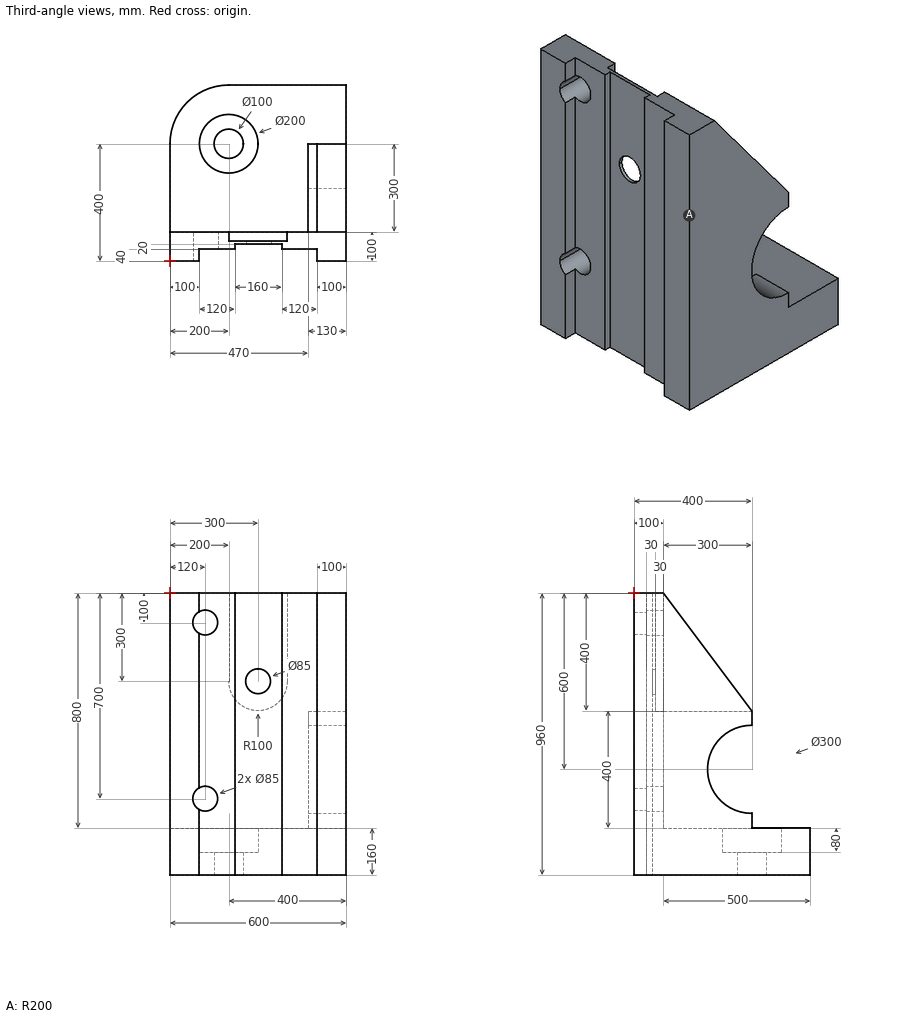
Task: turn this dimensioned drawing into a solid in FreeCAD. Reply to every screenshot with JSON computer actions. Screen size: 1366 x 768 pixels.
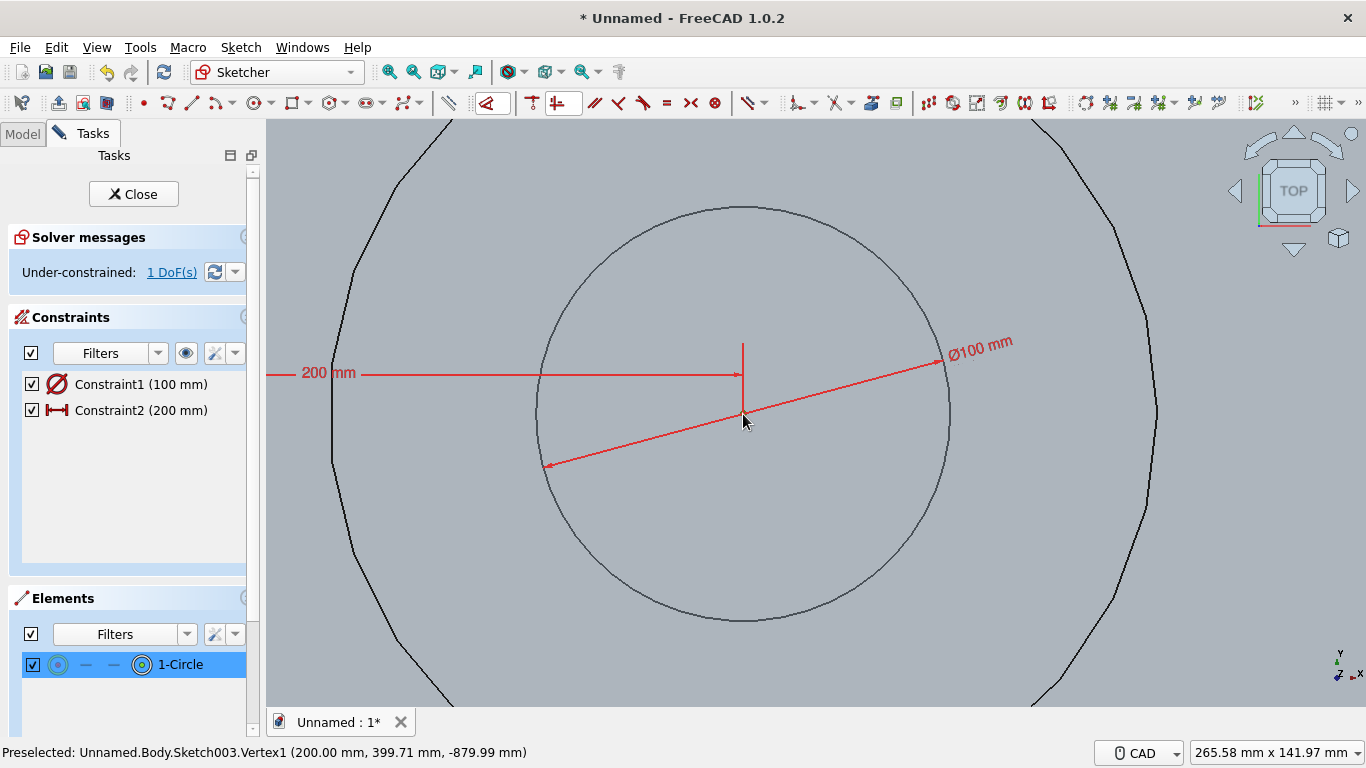
{"action": "left_click", "coordinate": [504, 104]}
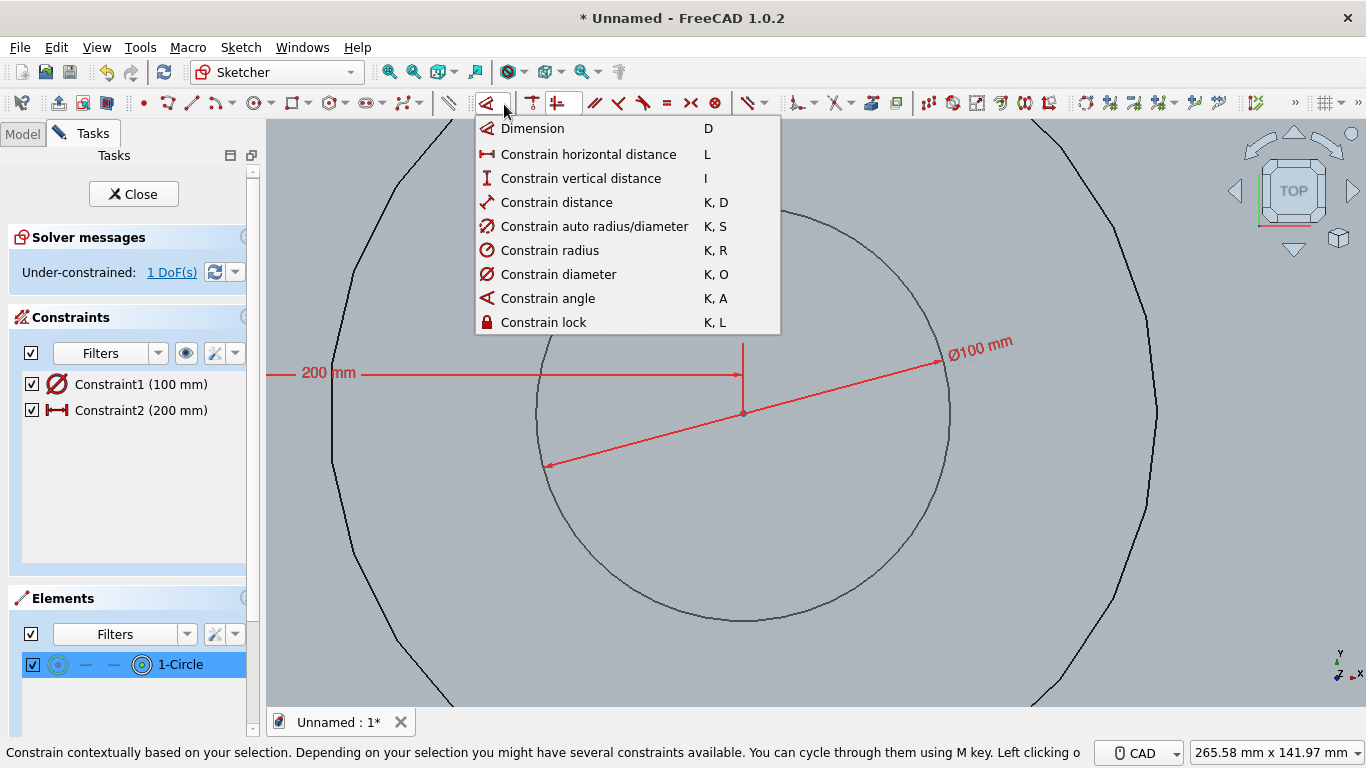
{"action": "left_click", "coordinate": [628, 178]}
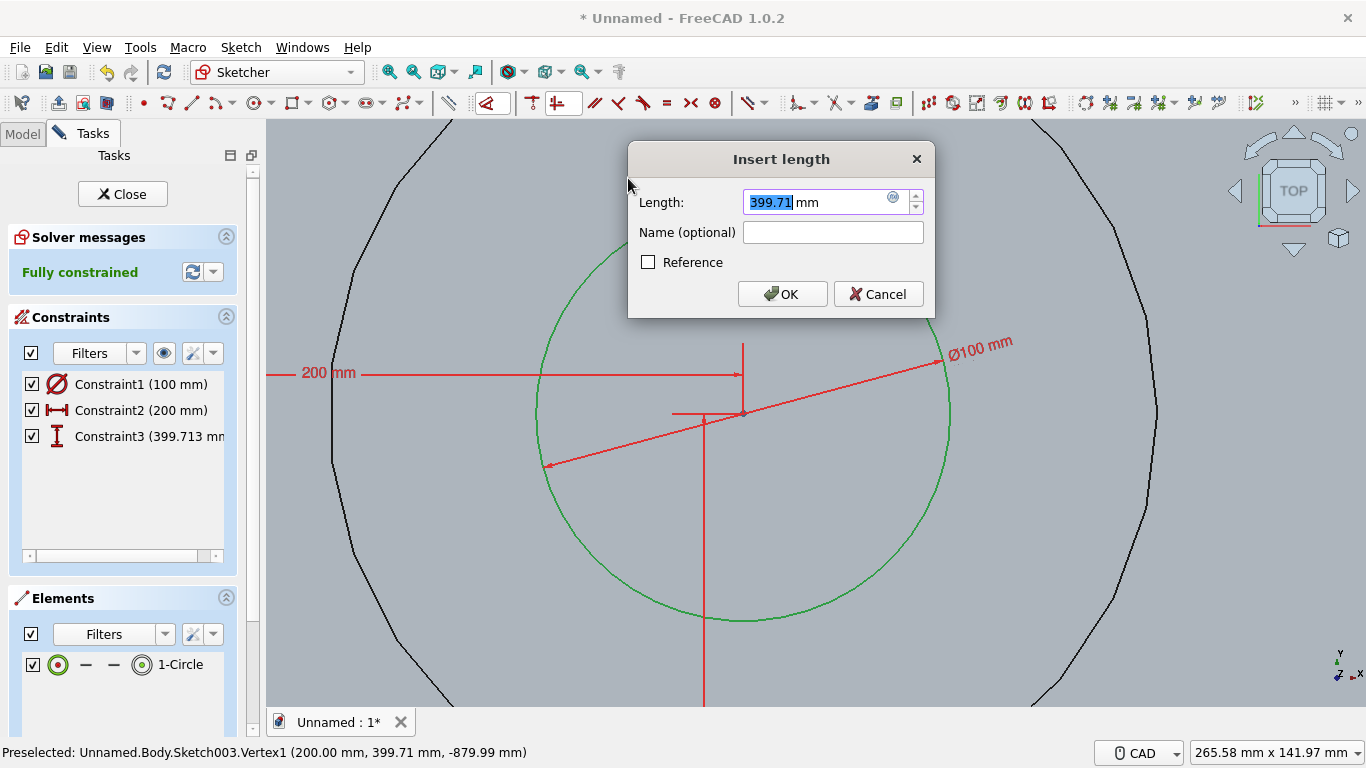
{"action": "type", "text": "400"}
{"action": "key", "text": "Return"}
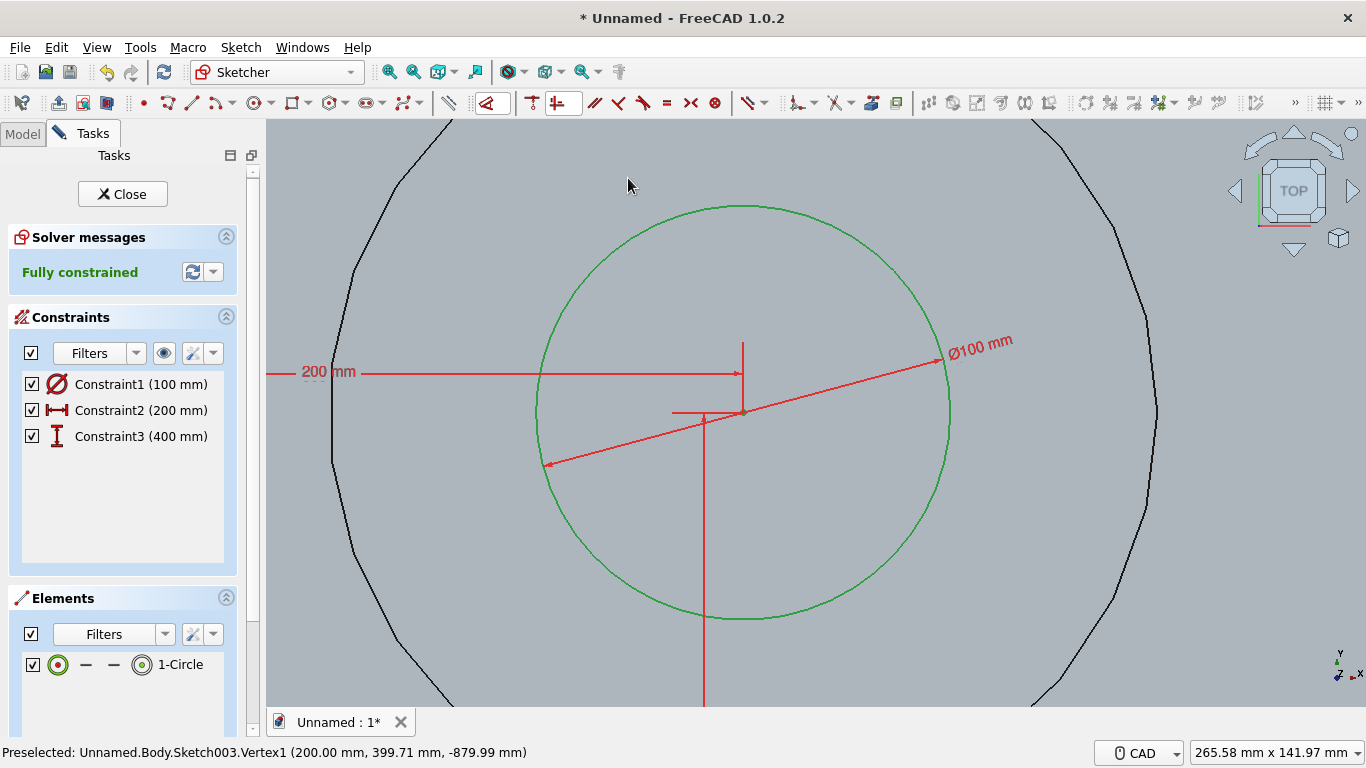
{"action": "left_click", "coordinate": [123, 194]}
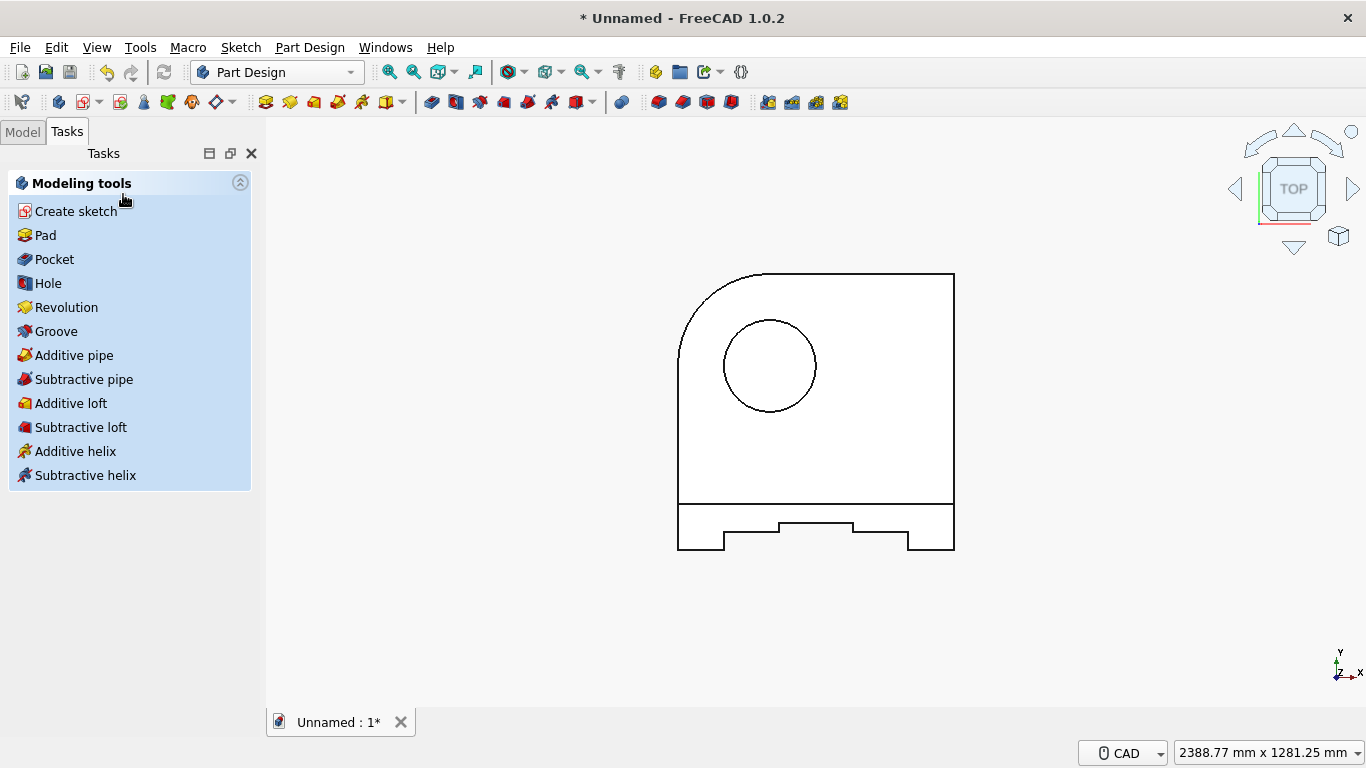
{"action": "left_click", "coordinate": [432, 102]}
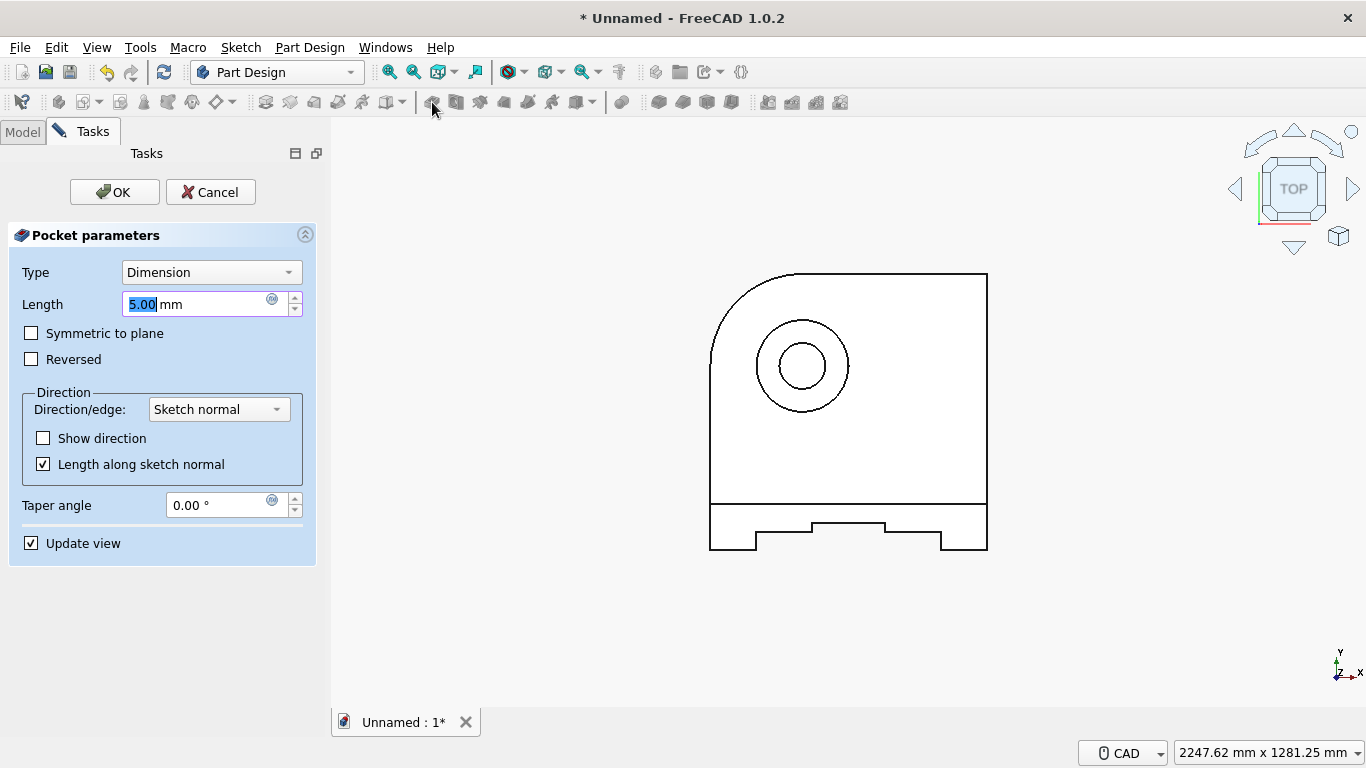
{"action": "left_click", "coordinate": [212, 272]}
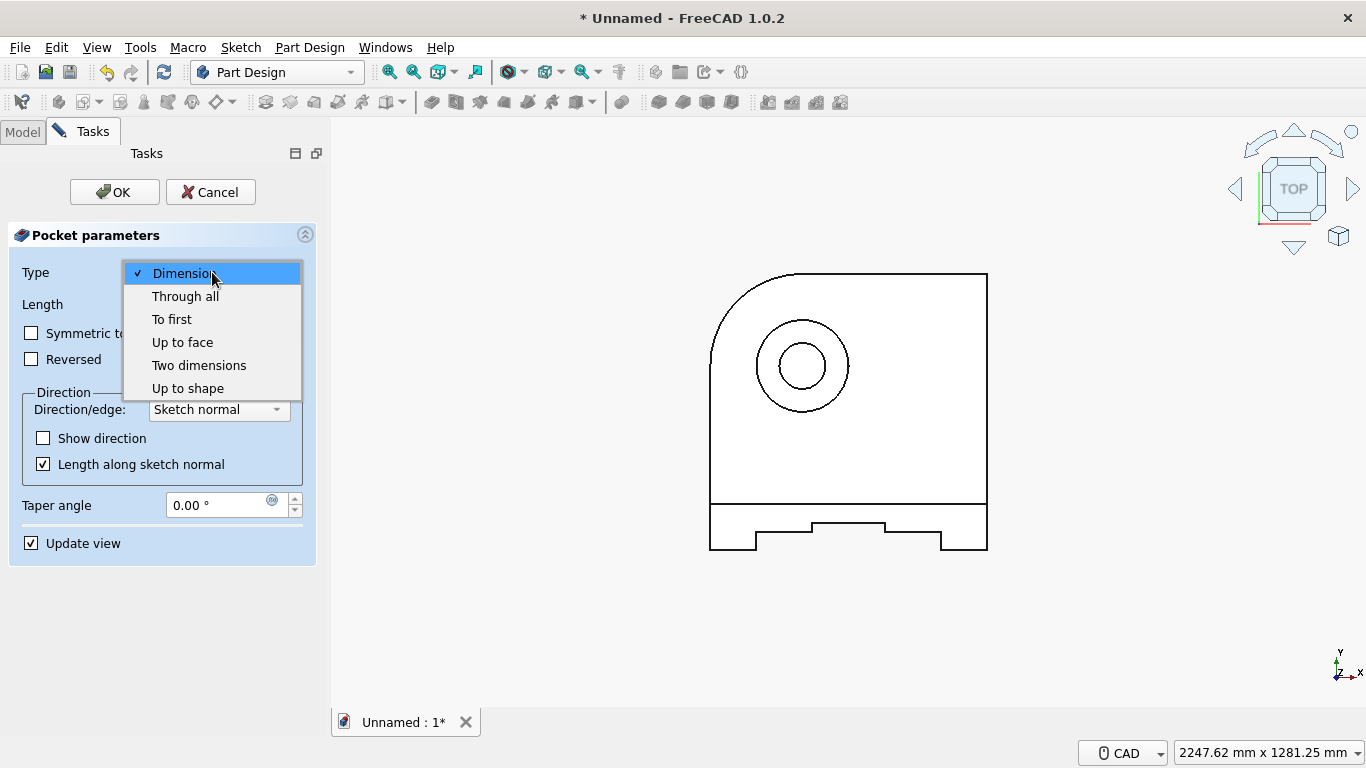
{"action": "left_click", "coordinate": [212, 296]}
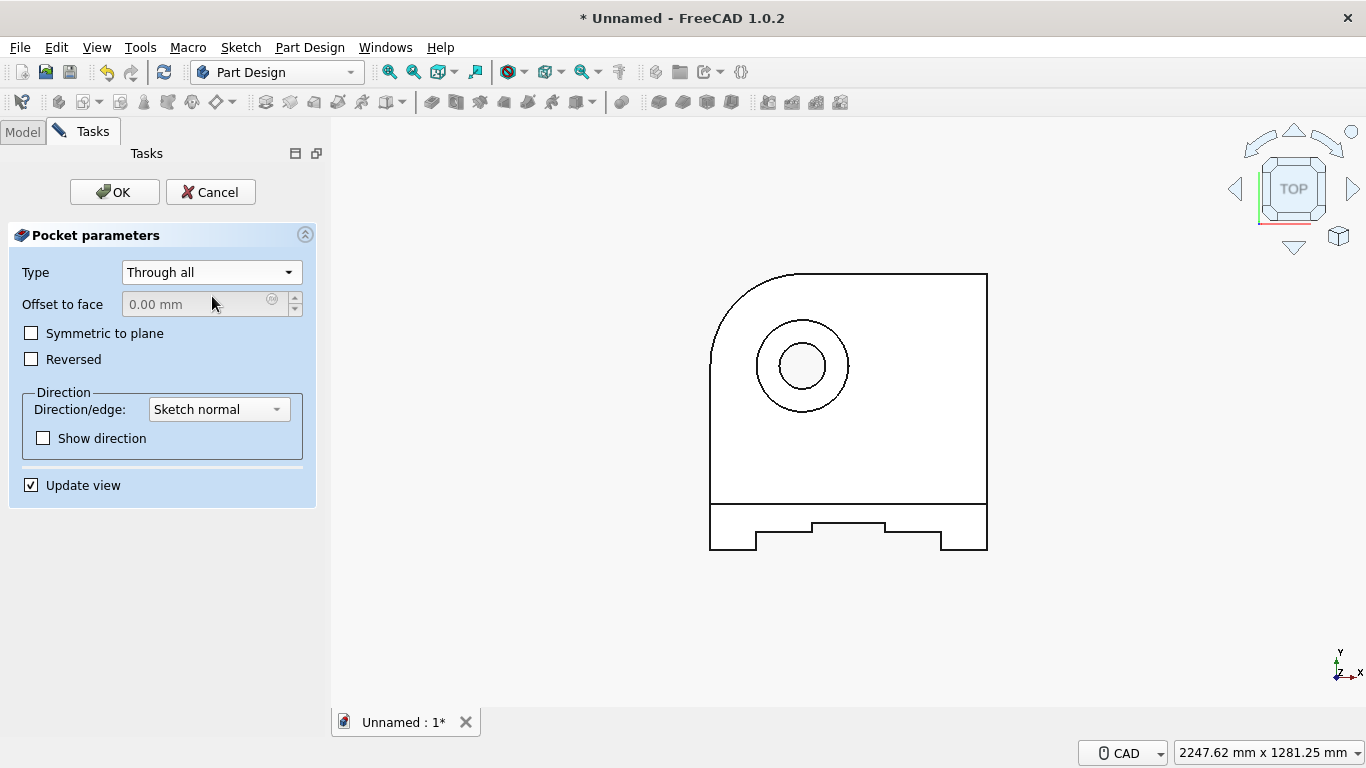
{"action": "left_click", "coordinate": [115, 192]}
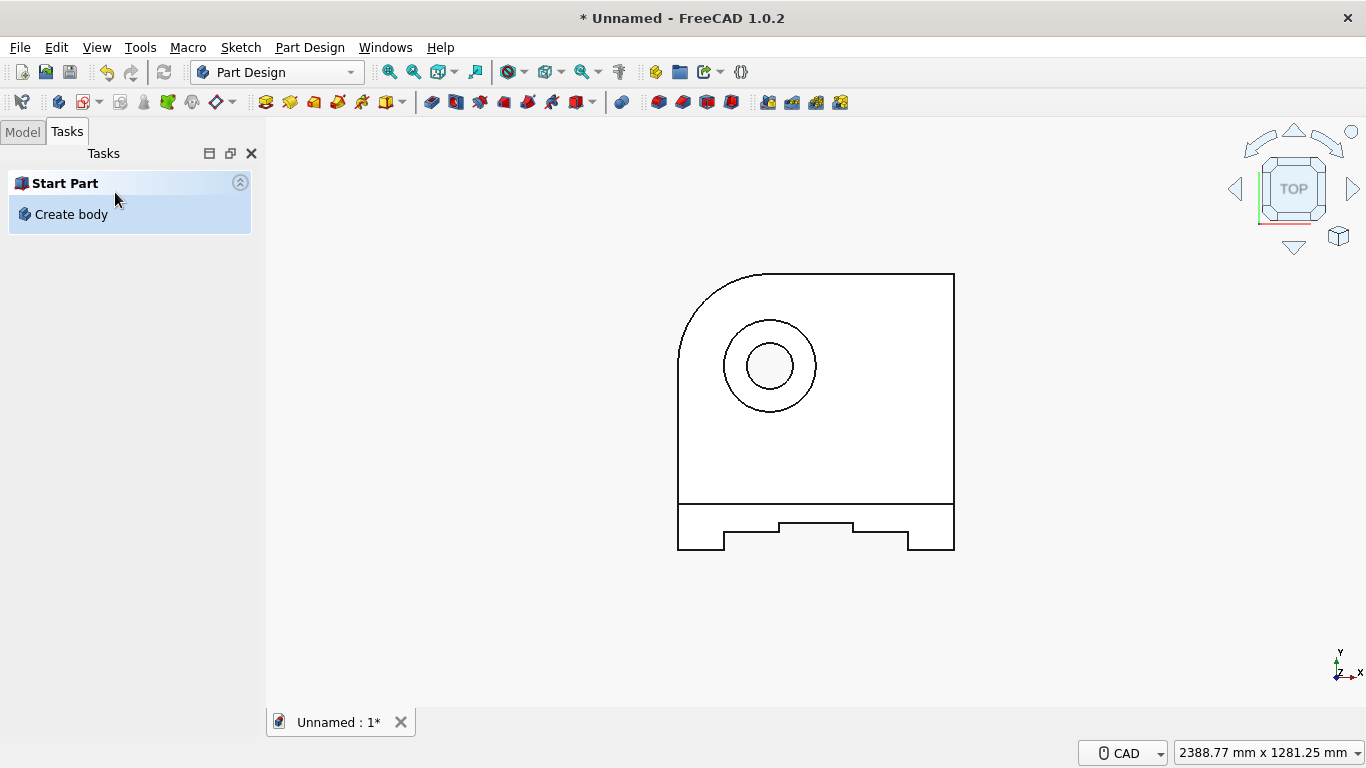
{"action": "key", "text": "4"}